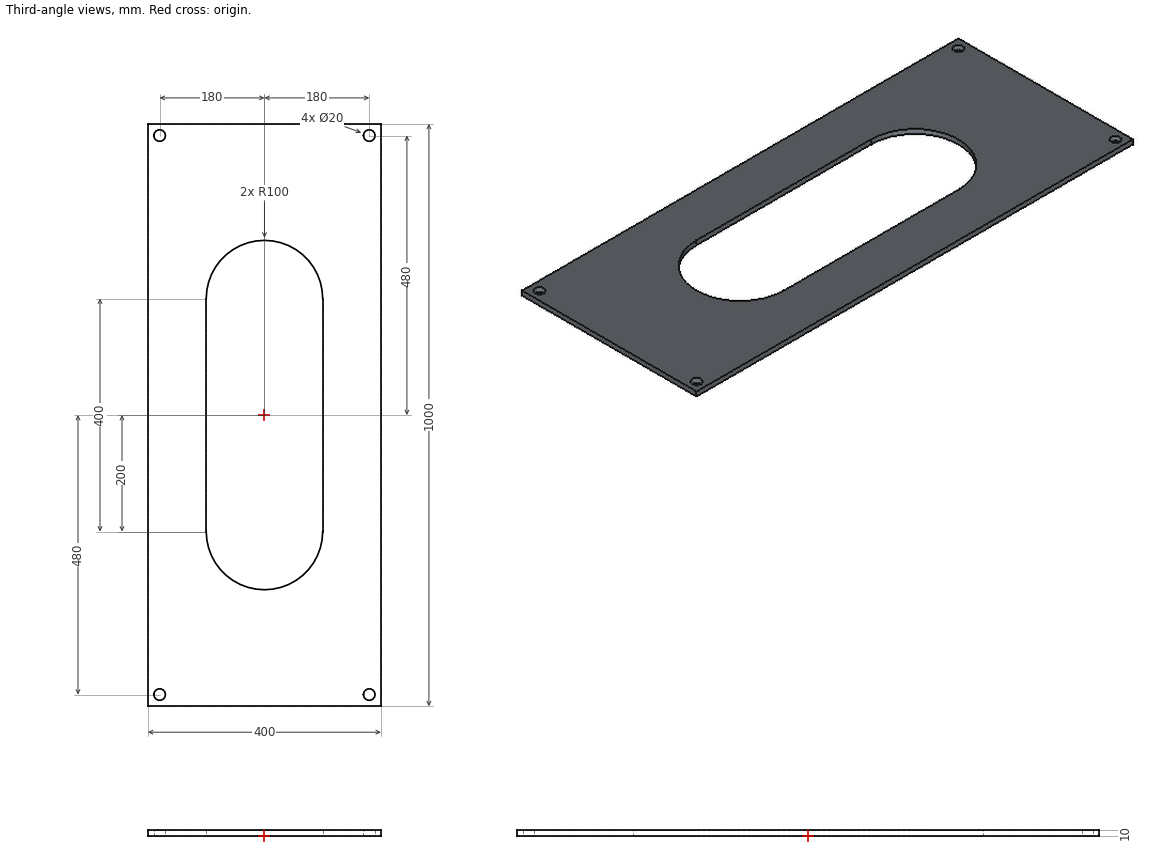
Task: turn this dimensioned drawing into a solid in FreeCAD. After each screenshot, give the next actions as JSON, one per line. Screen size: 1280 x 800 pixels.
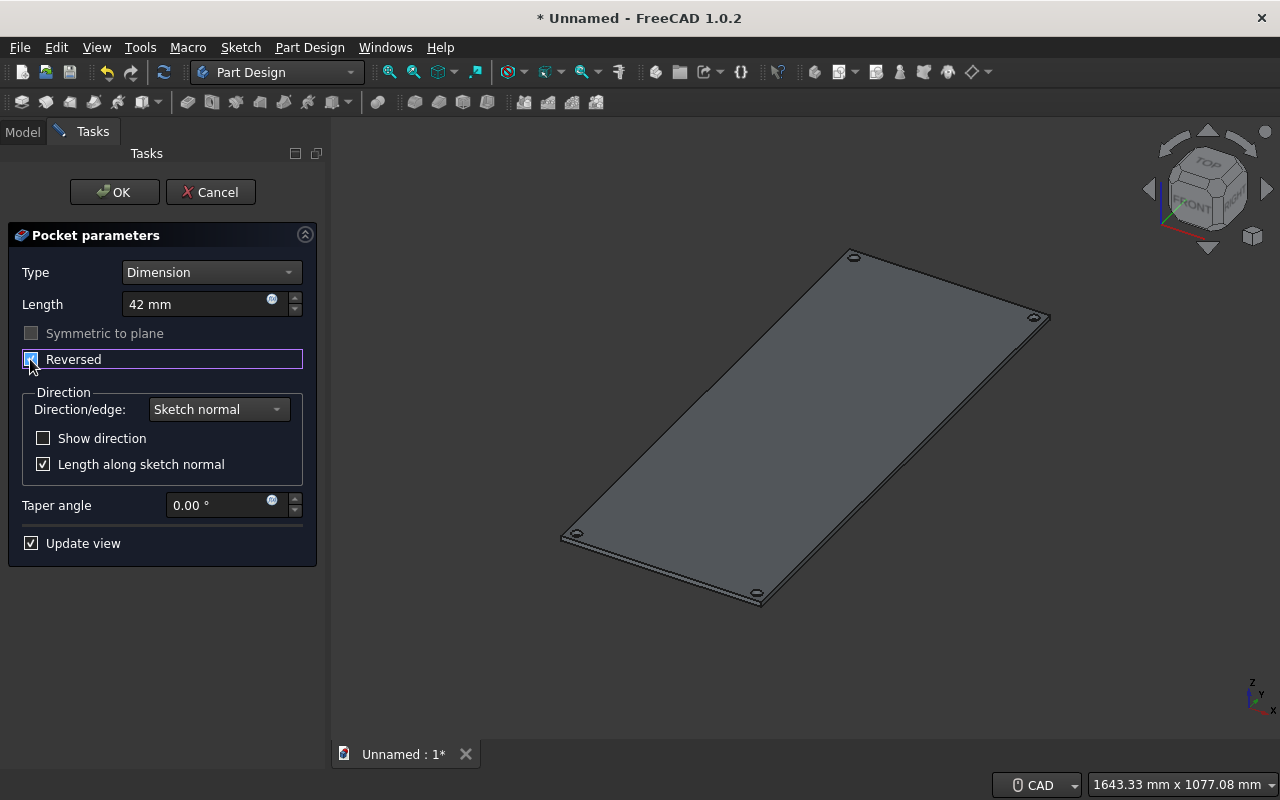
{"action": "left_click", "coordinate": [115, 192]}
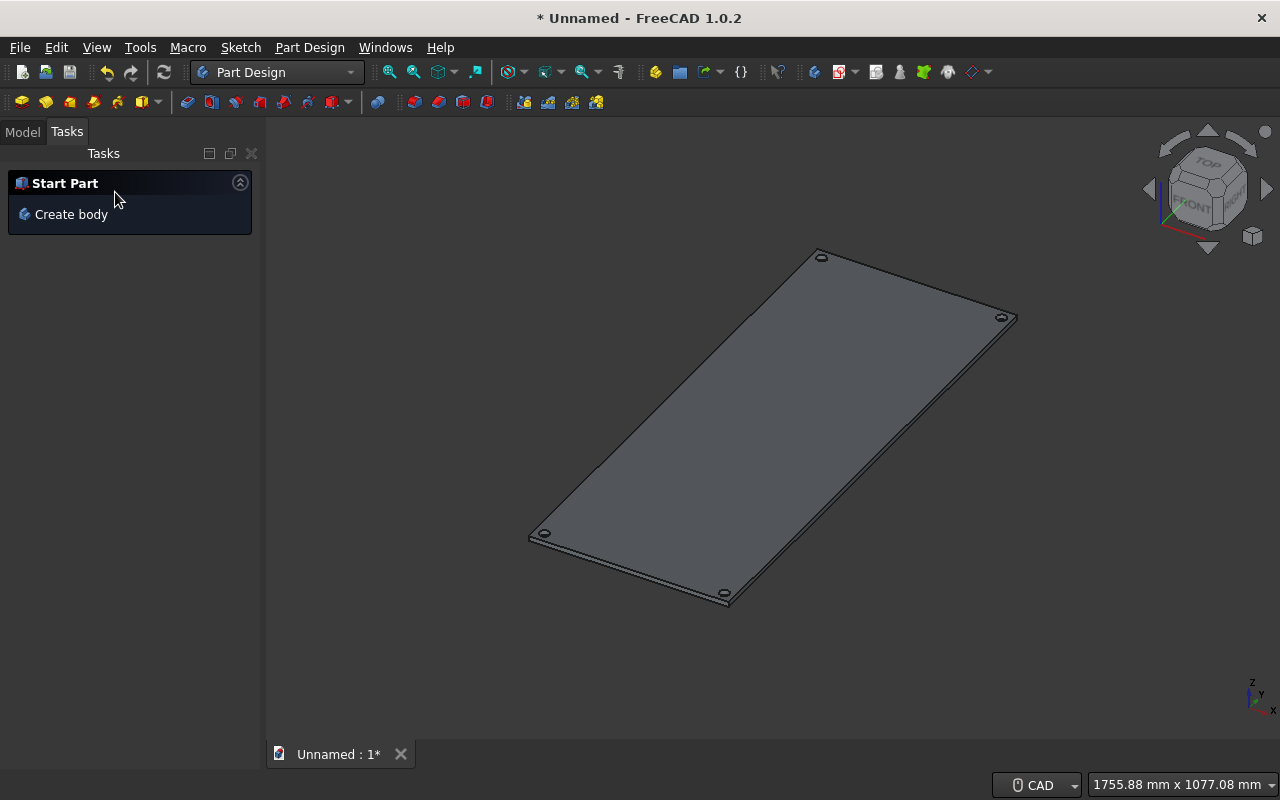
{"action": "left_click", "coordinate": [855, 343]}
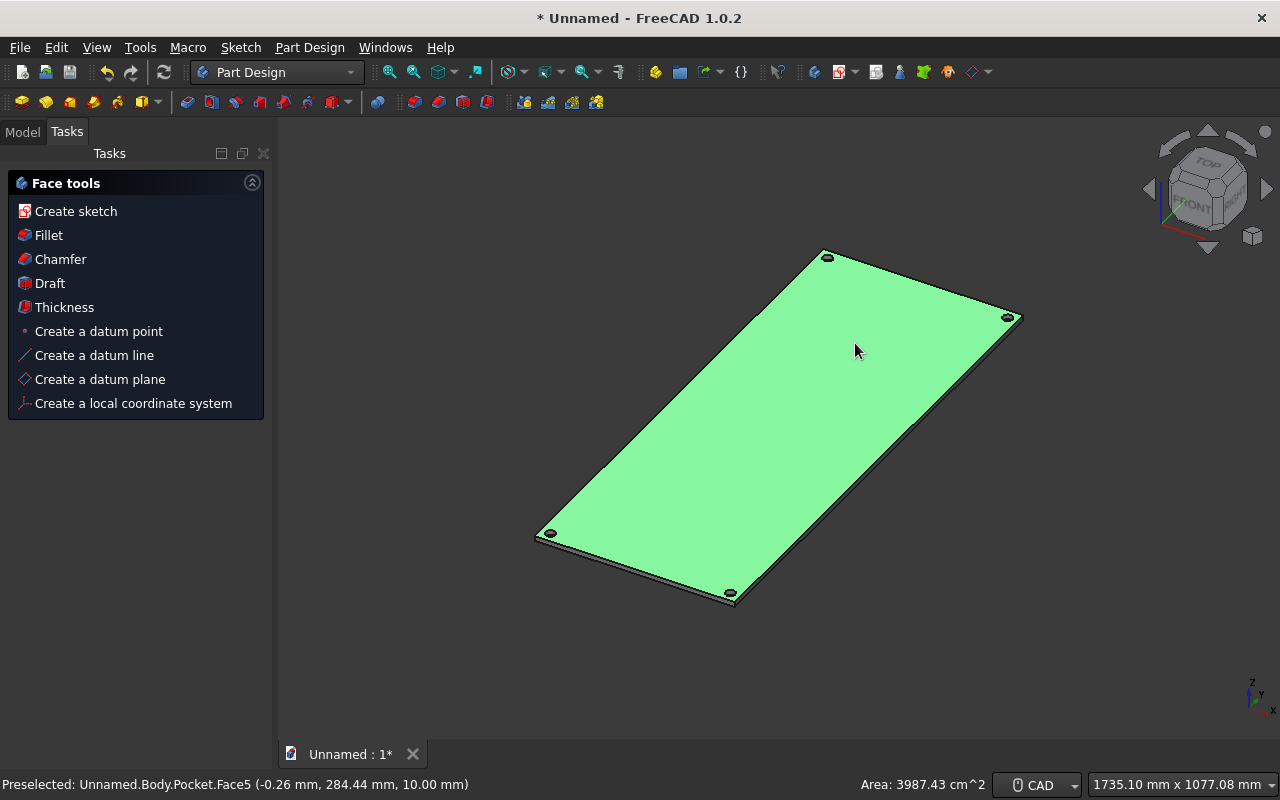
{"action": "left_click", "coordinate": [840, 72]}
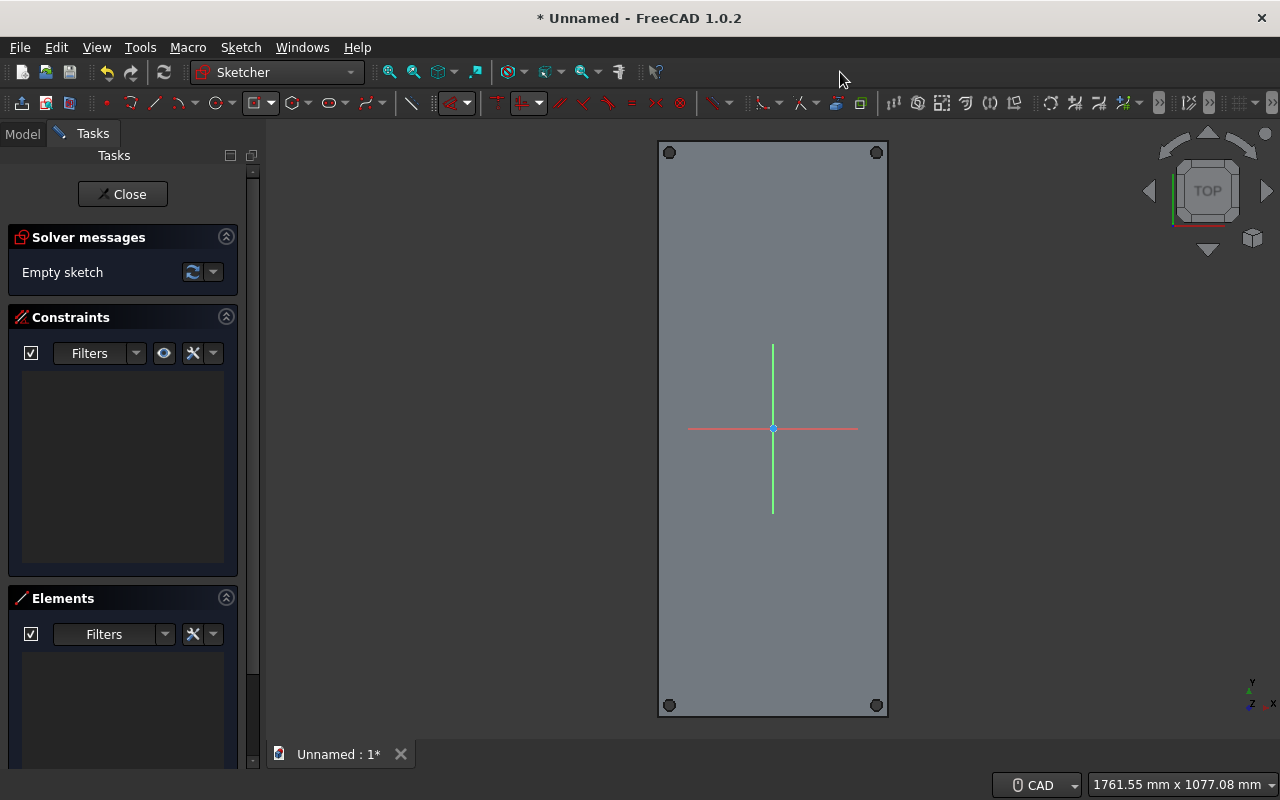
{"action": "left_click", "coordinate": [330, 104]}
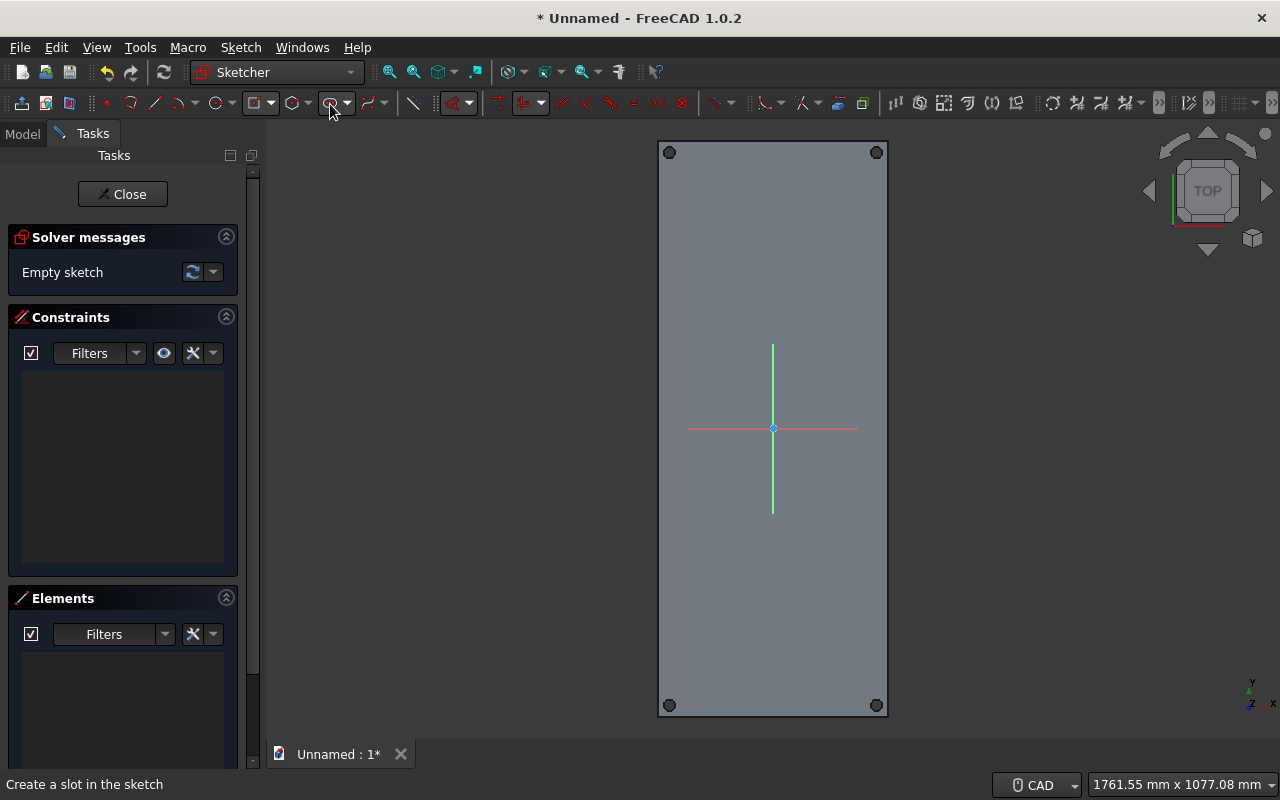
{"action": "left_click", "coordinate": [773, 544]}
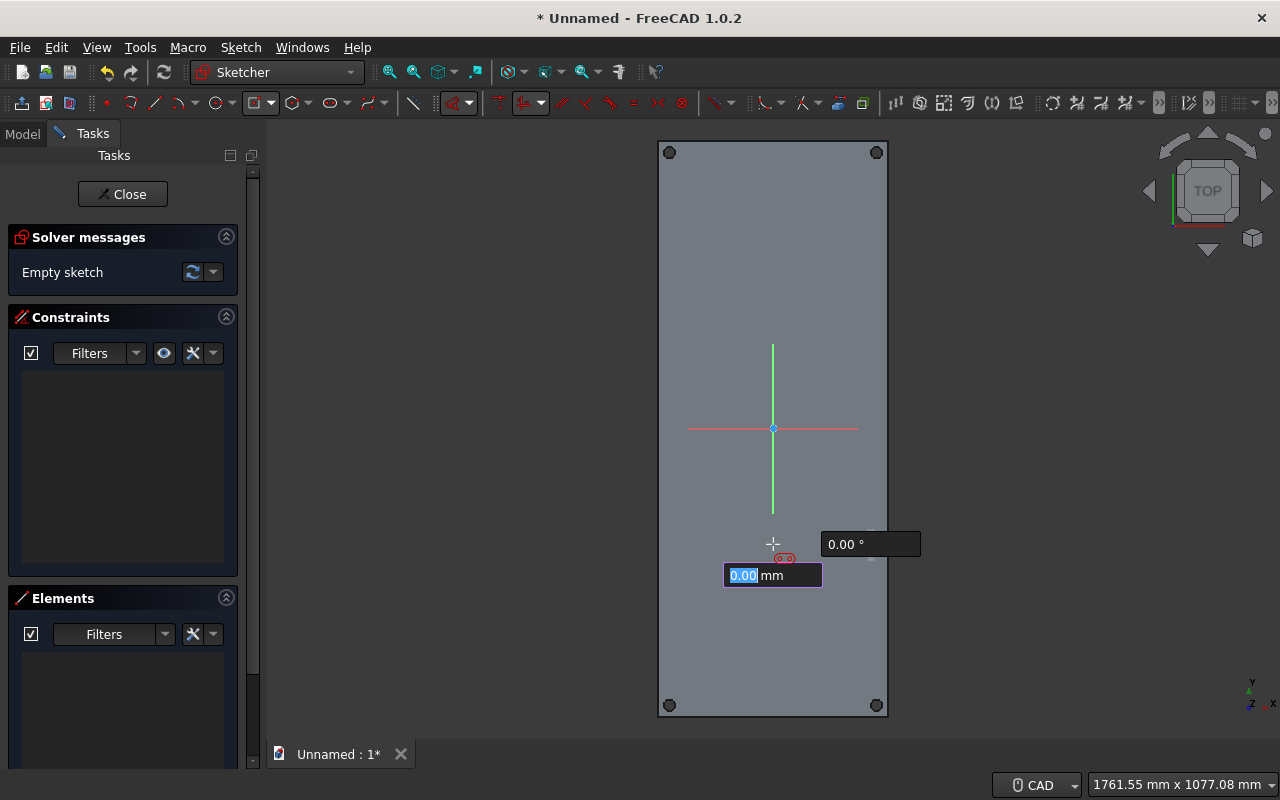
{"action": "left_click", "coordinate": [782, 314]}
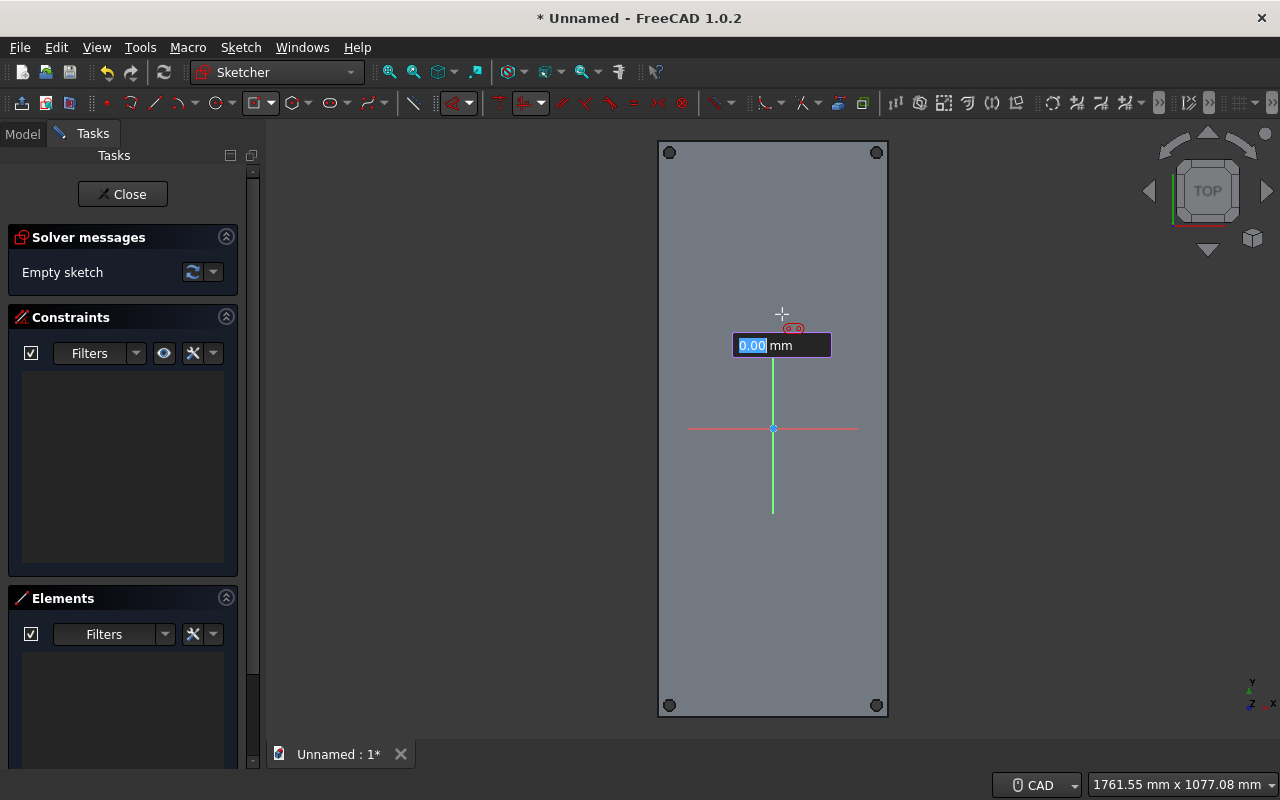
{"action": "left_click", "coordinate": [831, 464]}
{"action": "key", "text": "Escape"}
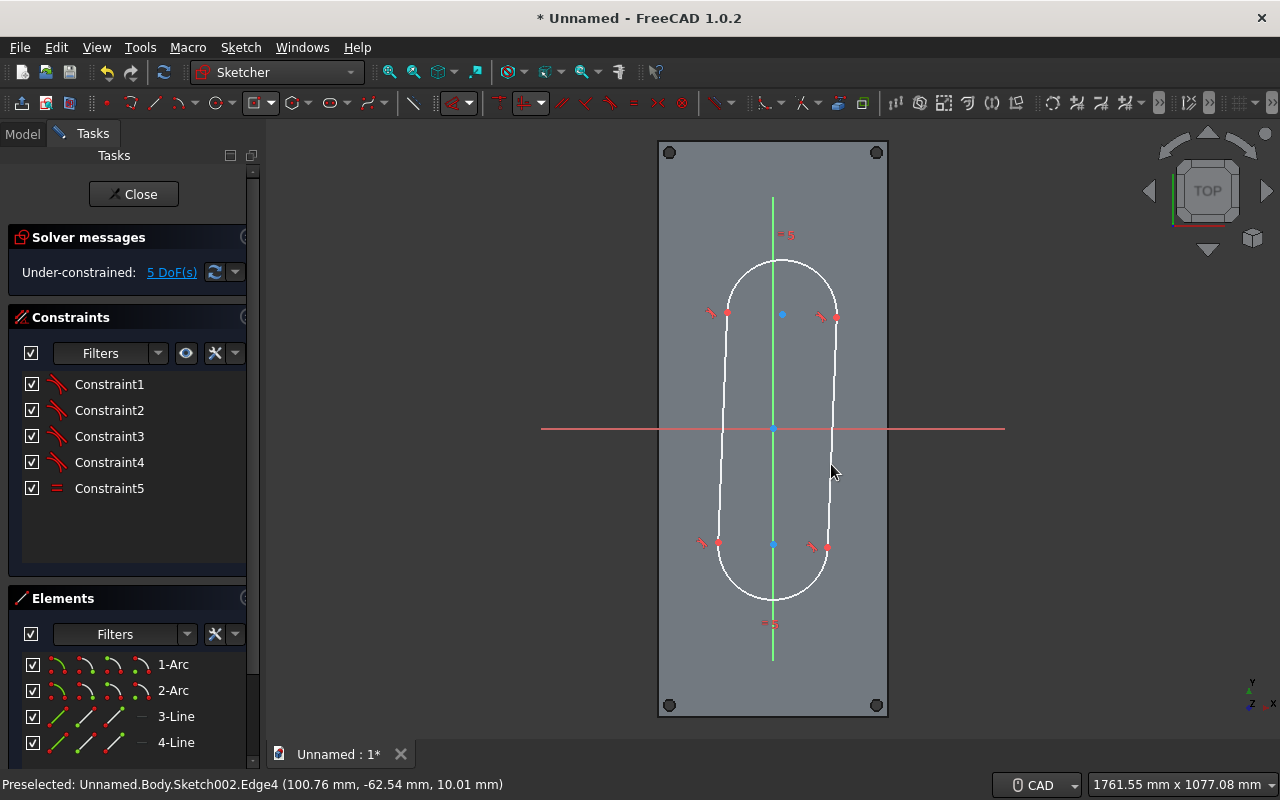
{"action": "left_click", "coordinate": [721, 474]}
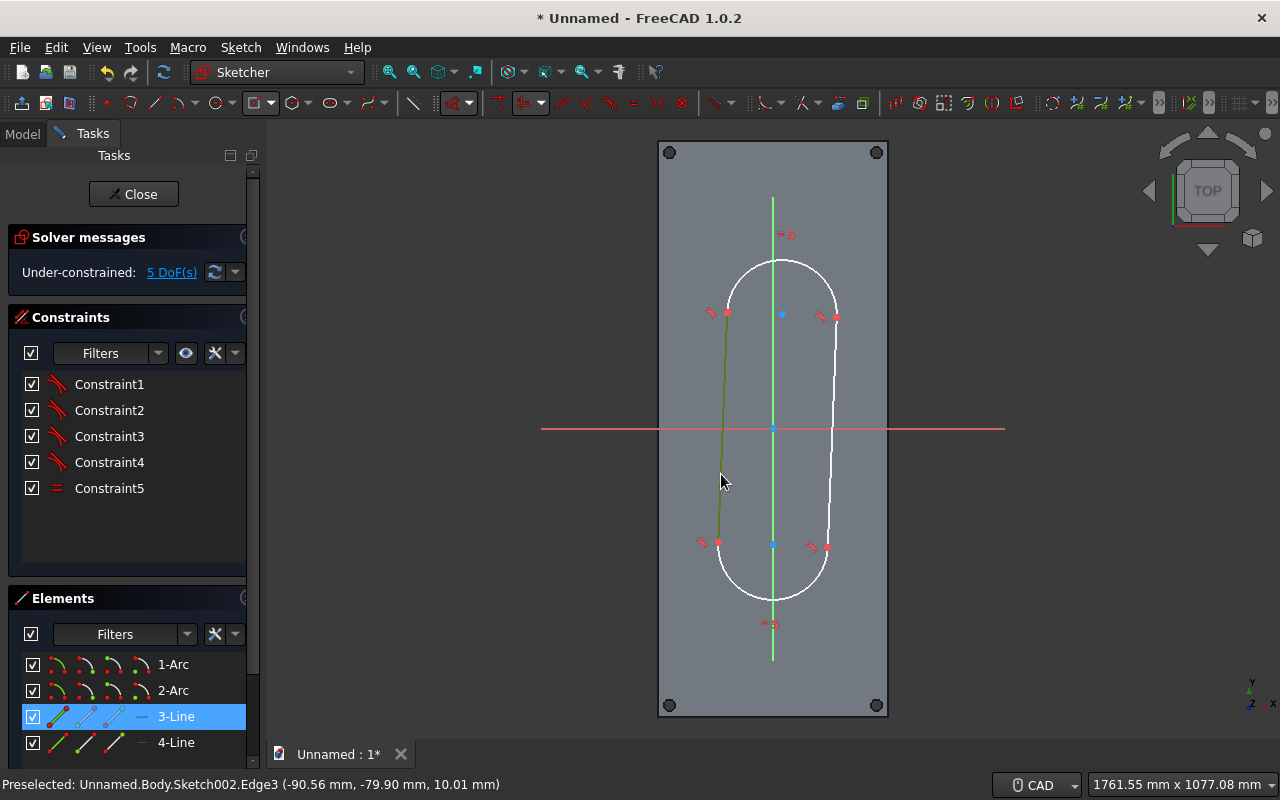
{"action": "key", "text": "v"}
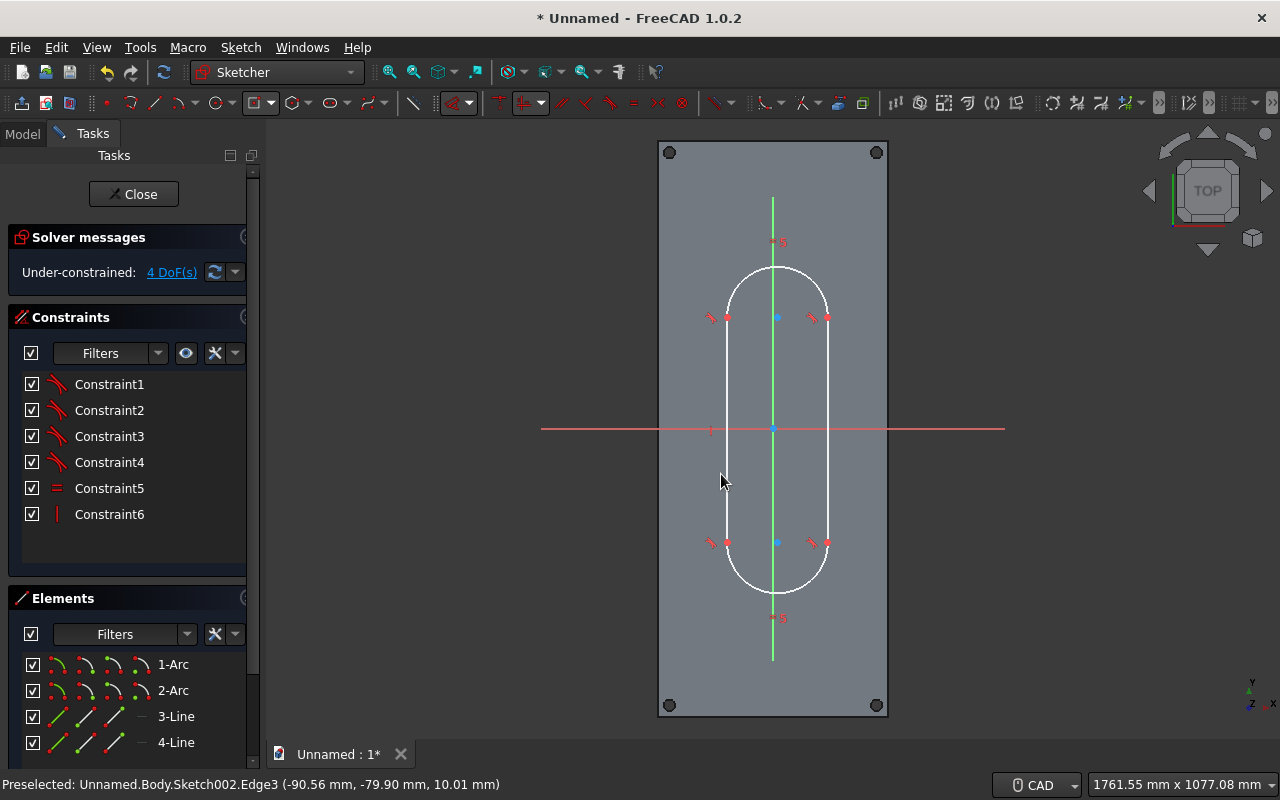
{"action": "left_click", "coordinate": [777, 543]}